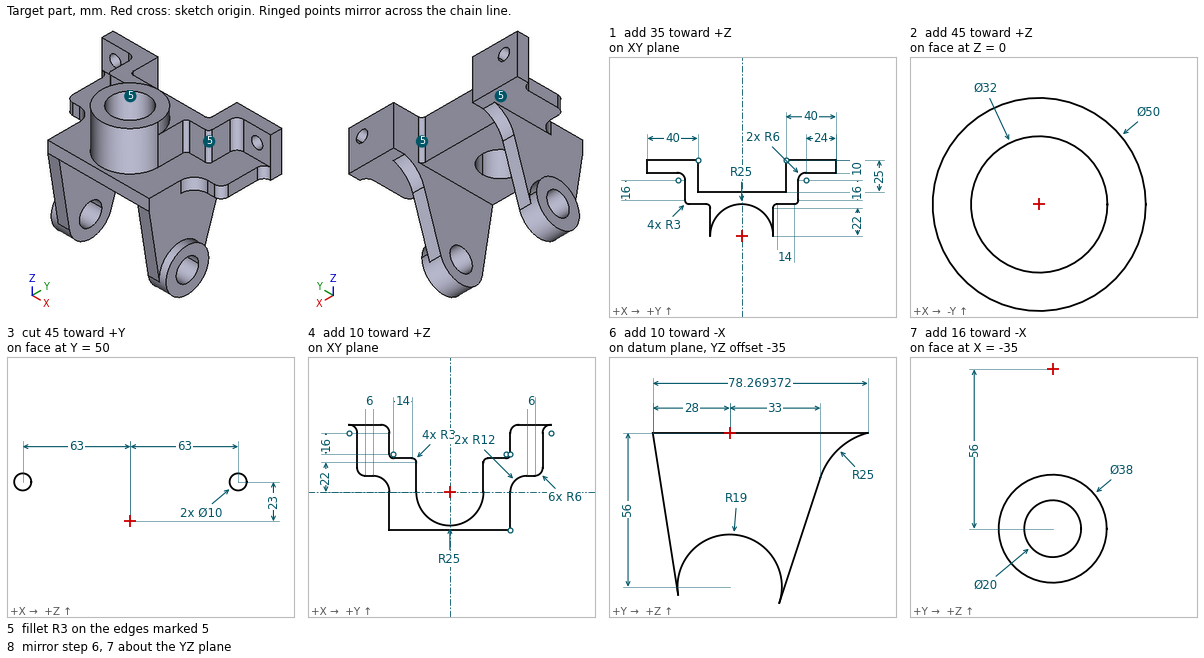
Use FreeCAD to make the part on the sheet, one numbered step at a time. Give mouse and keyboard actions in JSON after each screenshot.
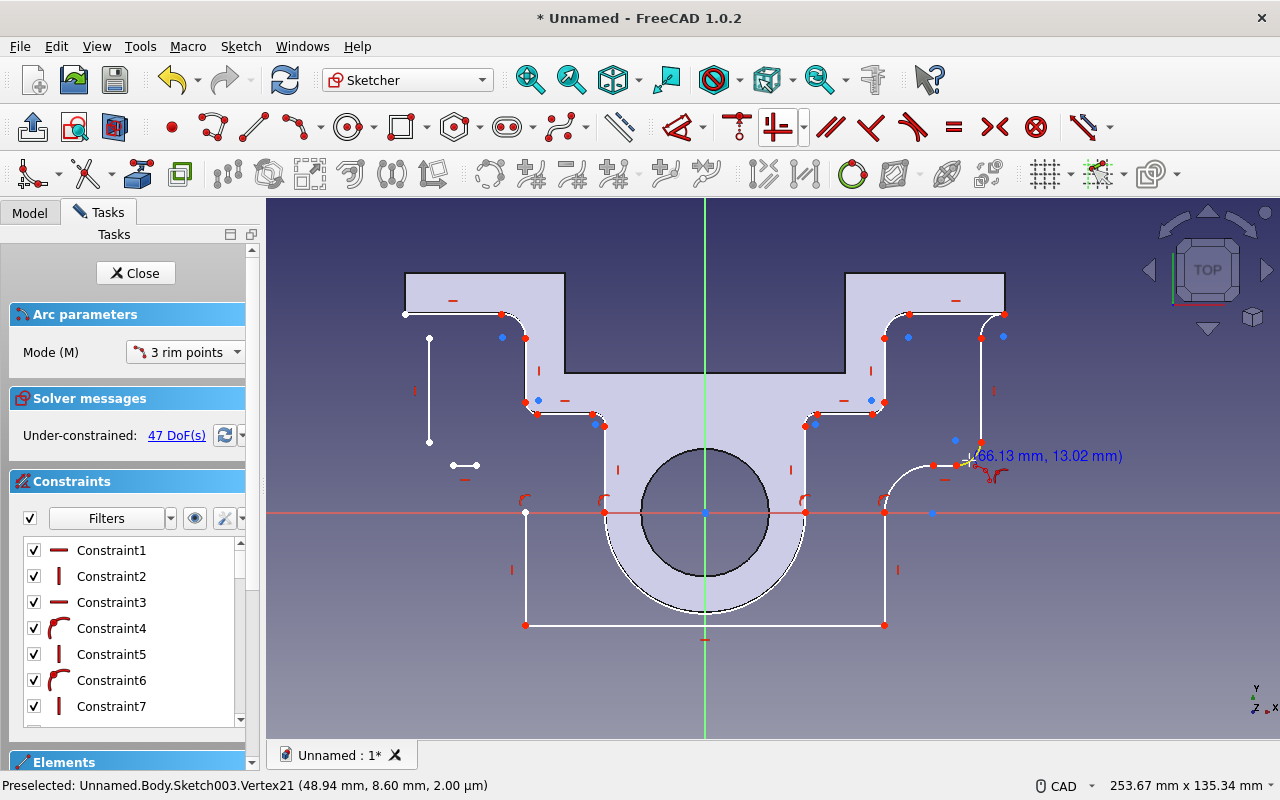
{"action": "left_click", "coordinate": [526, 513]}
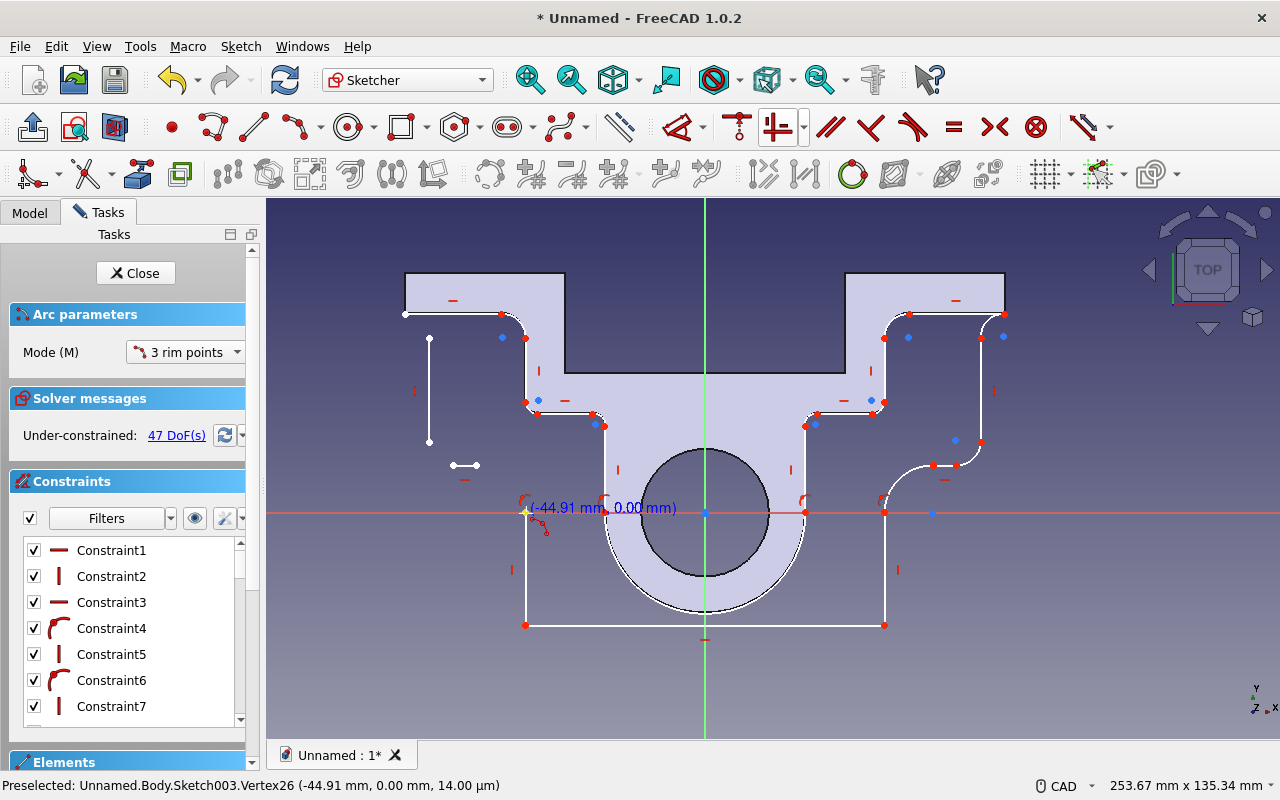
{"action": "scroll", "coordinate": [477, 465], "scroll_direction": "up", "scroll_amount": 2}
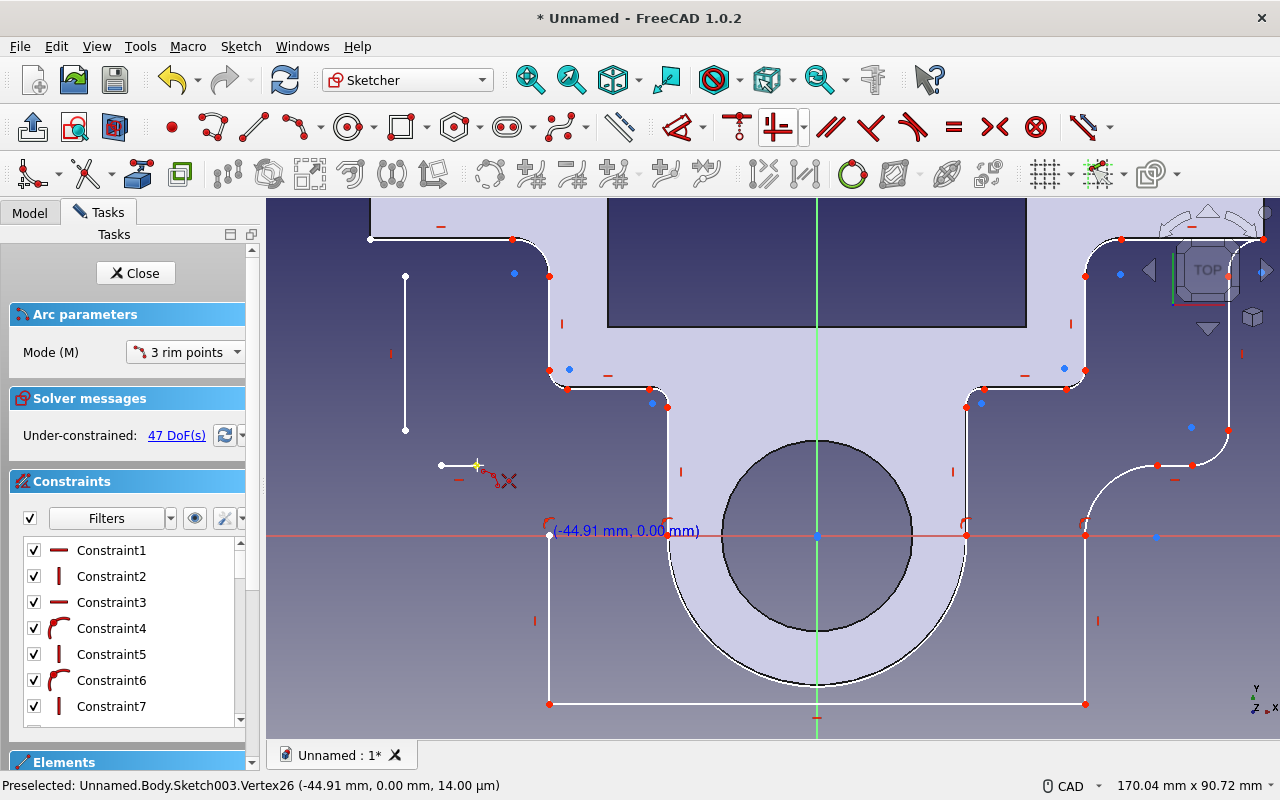
{"action": "left_click", "coordinate": [476, 466]}
{"action": "left_click", "coordinate": [528, 485]}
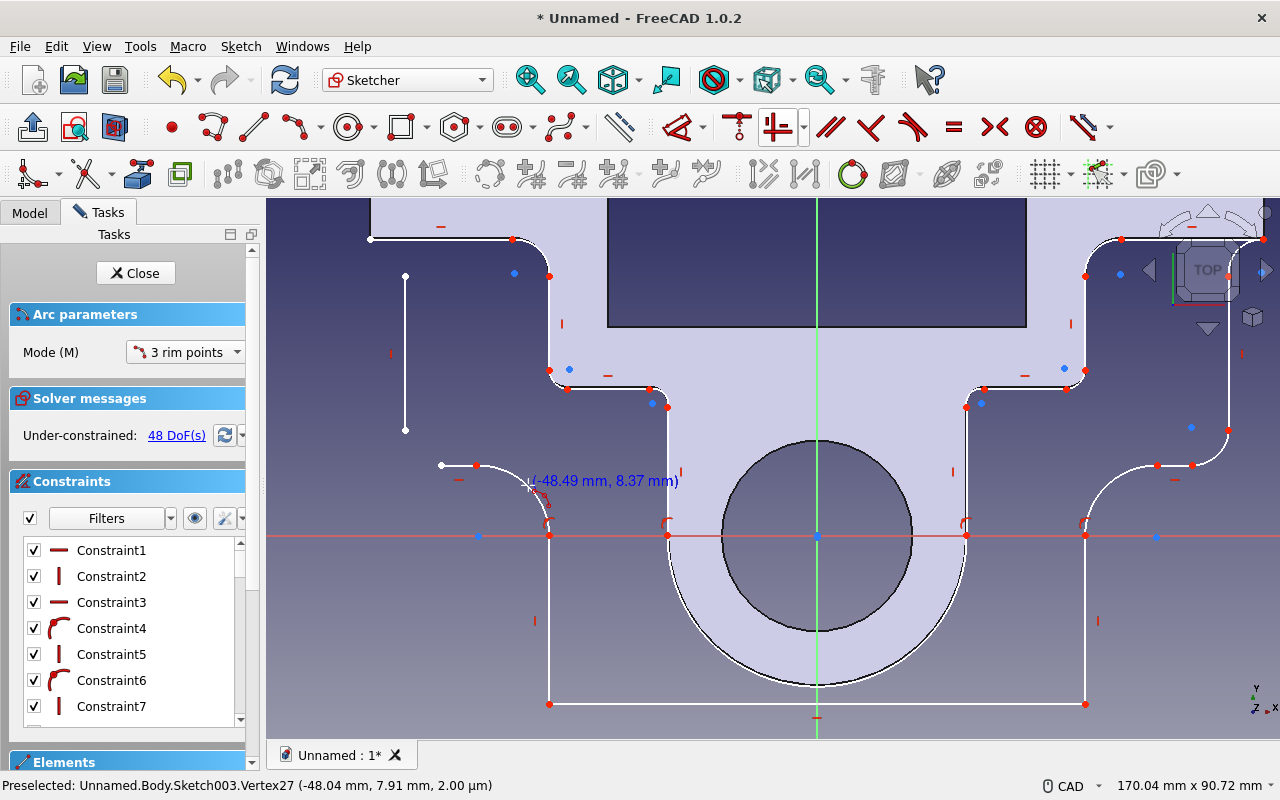
{"action": "left_click", "coordinate": [442, 466]}
{"action": "left_click", "coordinate": [405, 431]}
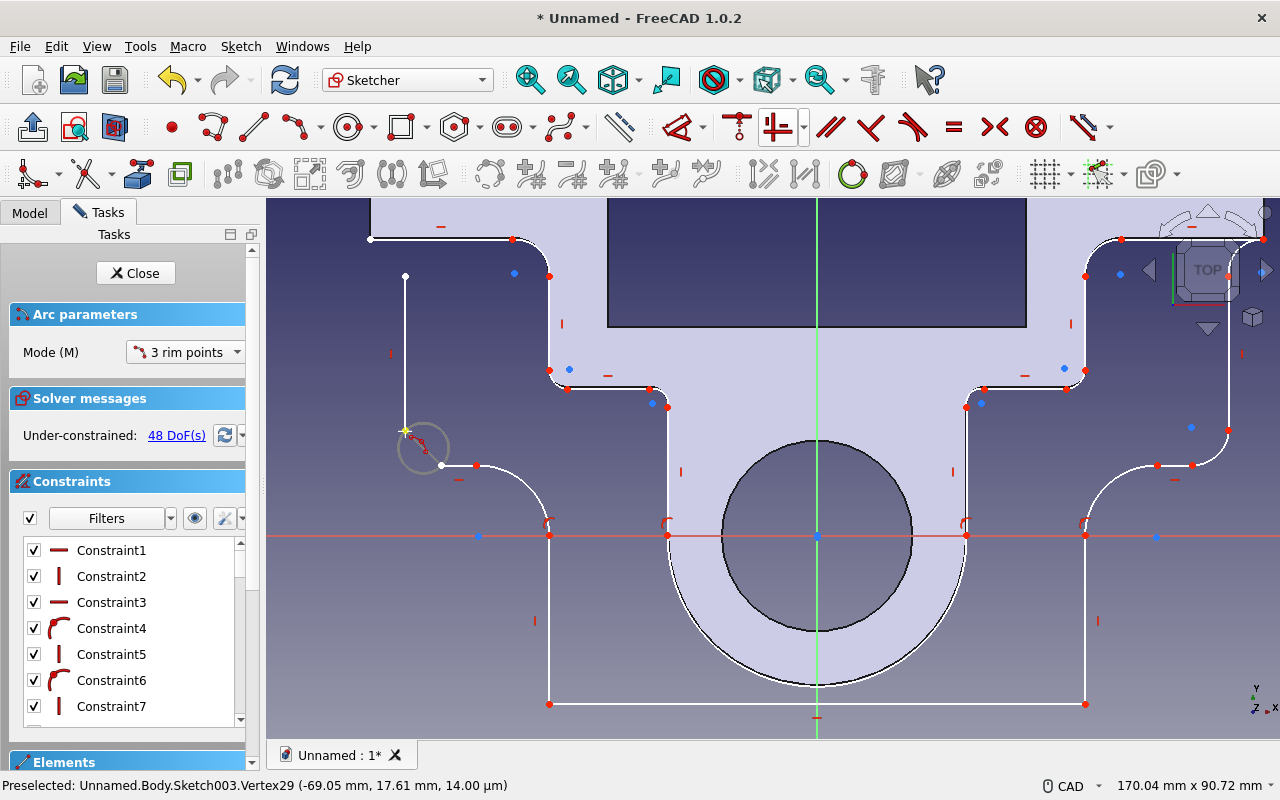
{"action": "scroll", "coordinate": [416, 454], "scroll_direction": "up", "scroll_amount": 3}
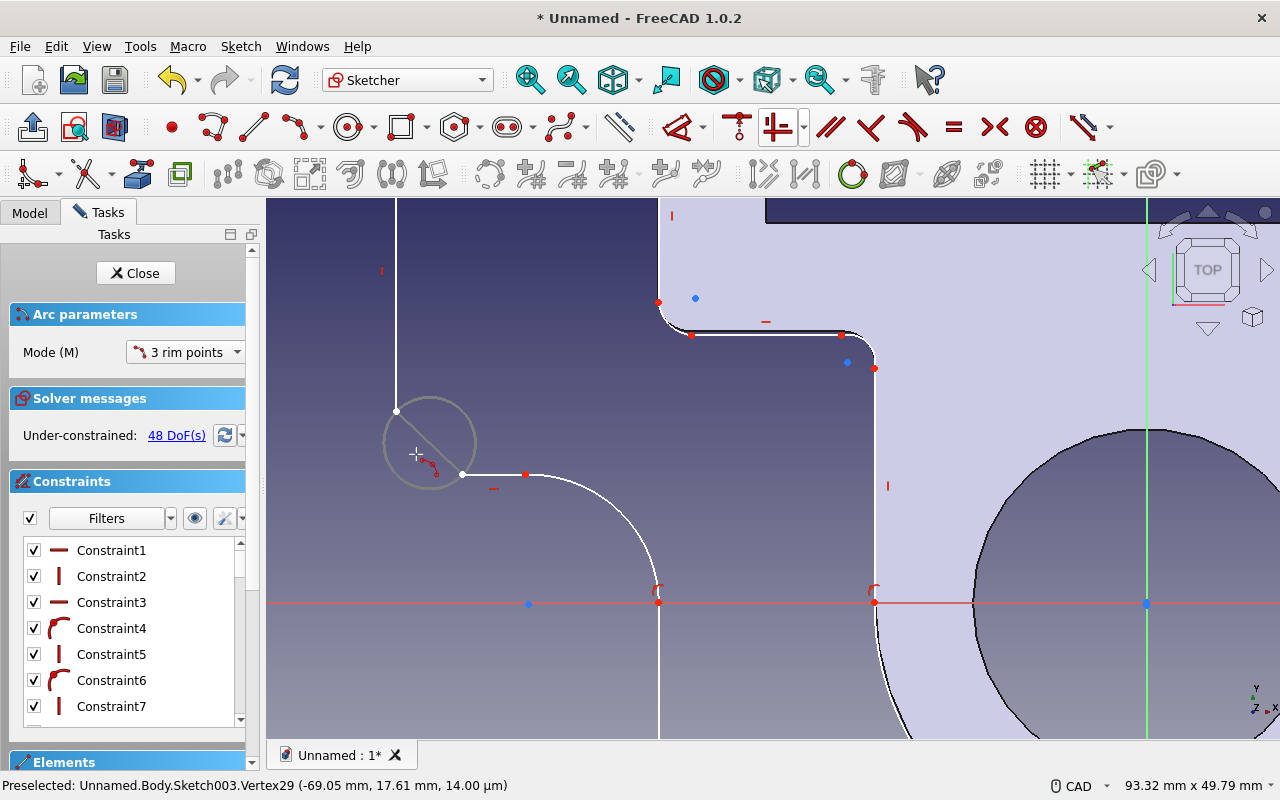
{"action": "left_click", "coordinate": [416, 453]}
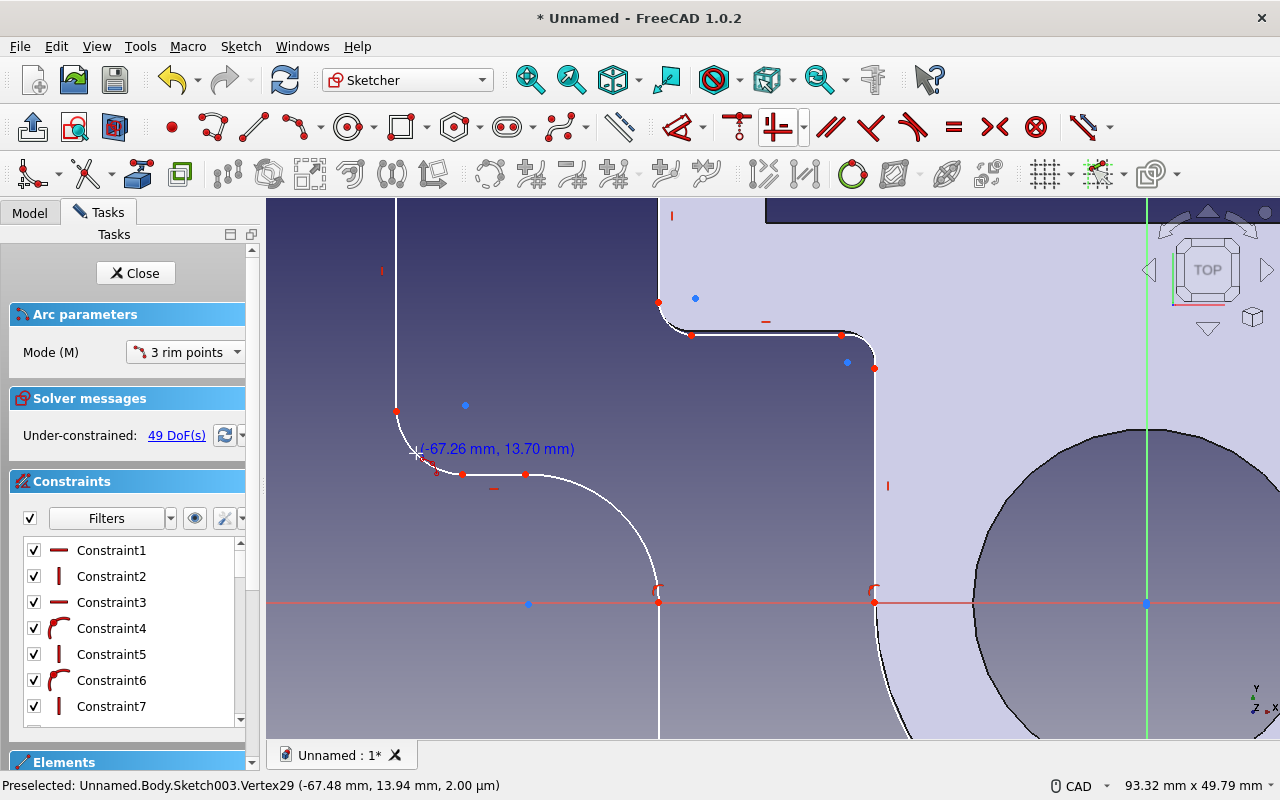
{"action": "scroll", "coordinate": [447, 460], "scroll_direction": "down", "scroll_amount": 5}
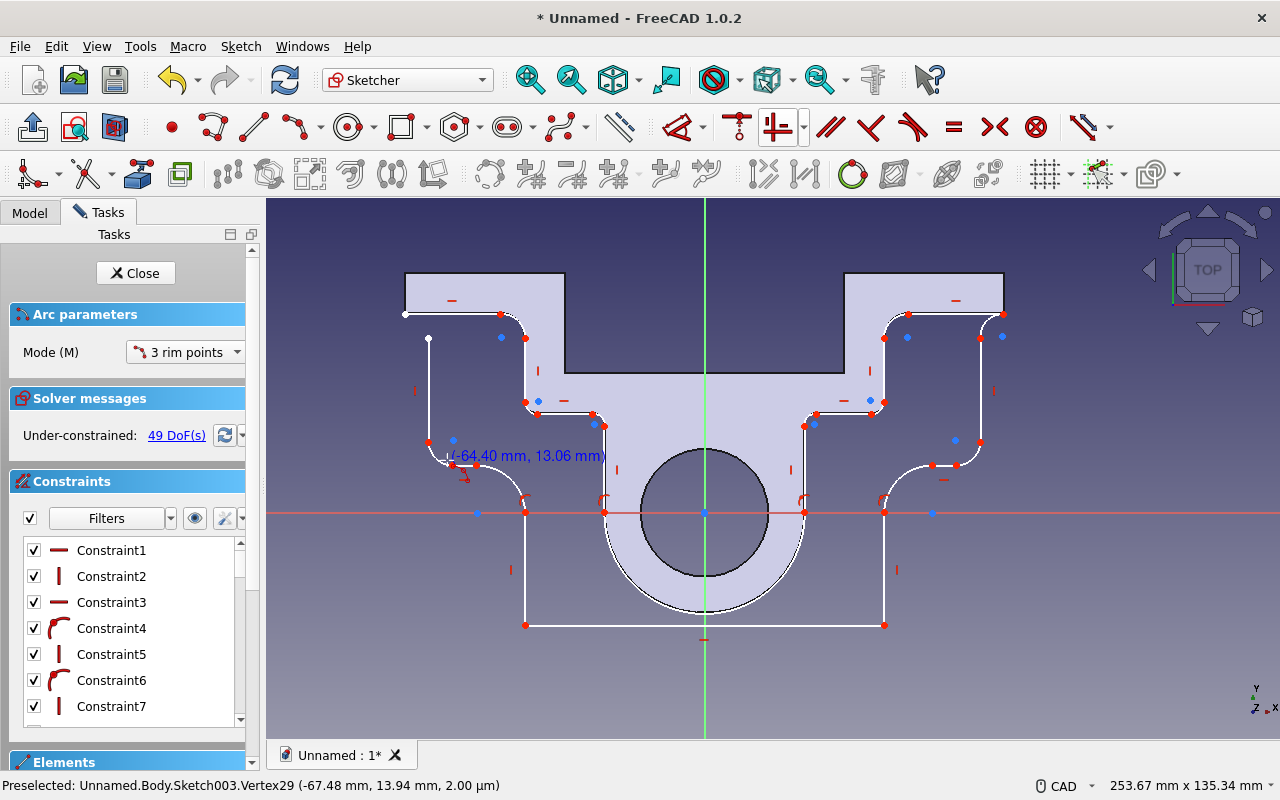
{"action": "left_click", "coordinate": [429, 339]}
{"action": "left_click", "coordinate": [405, 314]}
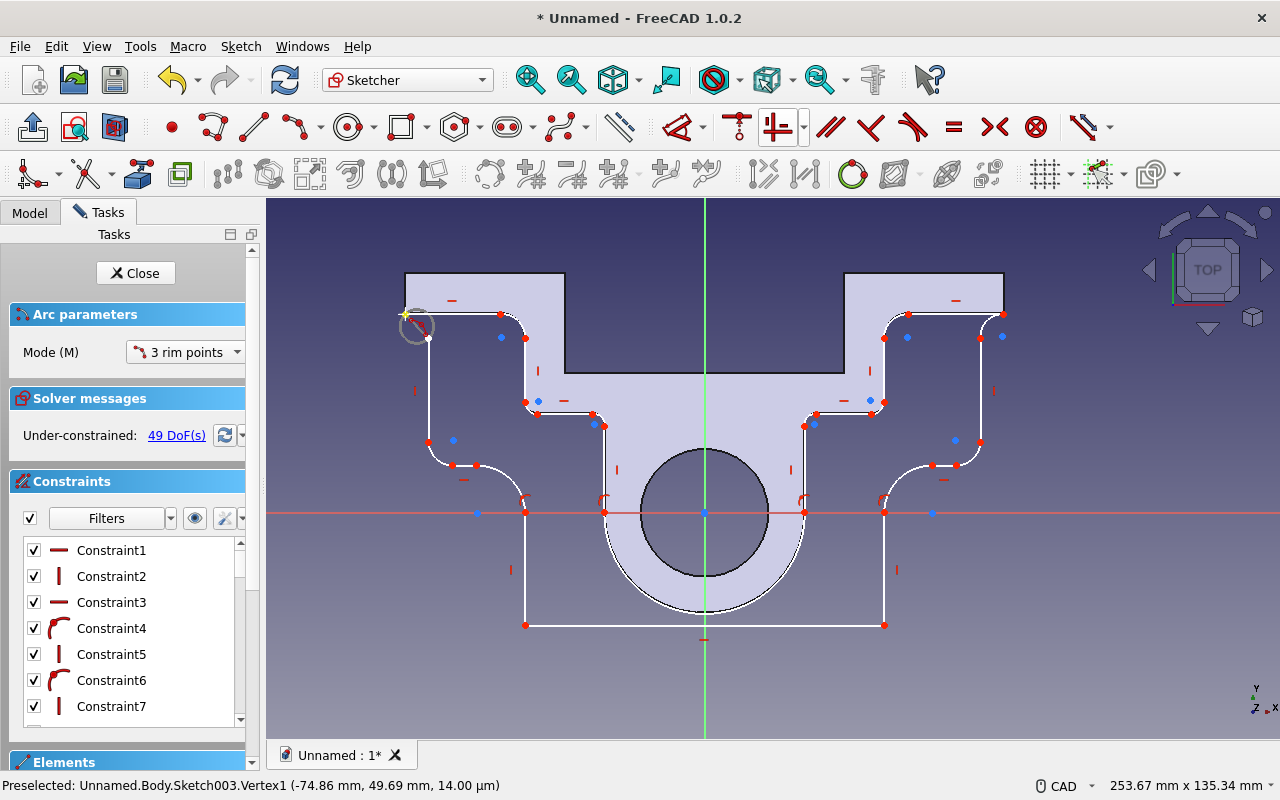
{"action": "scroll", "coordinate": [422, 320], "scroll_direction": "up", "scroll_amount": 5}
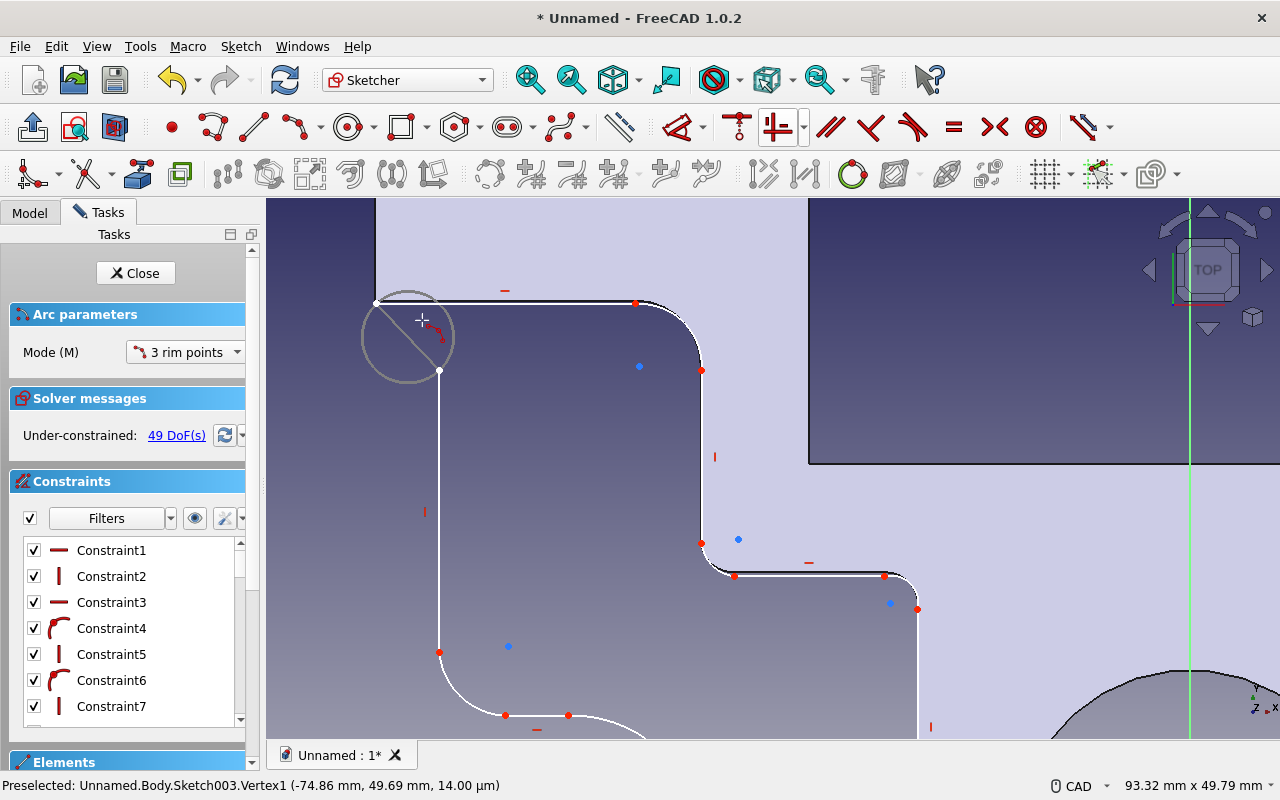
{"action": "left_click", "coordinate": [421, 320]}
{"action": "key", "text": "Escape"}